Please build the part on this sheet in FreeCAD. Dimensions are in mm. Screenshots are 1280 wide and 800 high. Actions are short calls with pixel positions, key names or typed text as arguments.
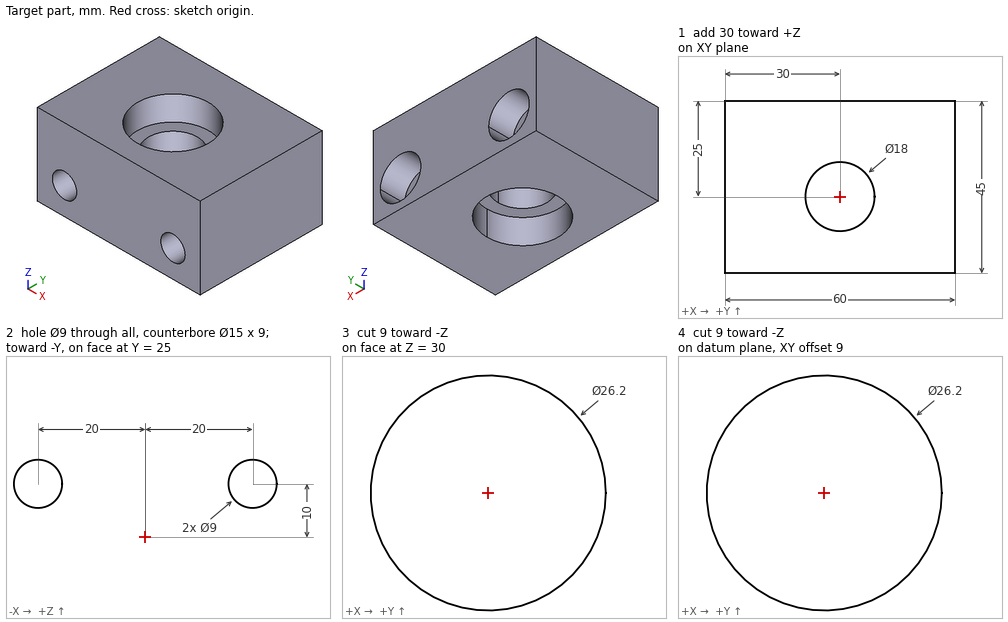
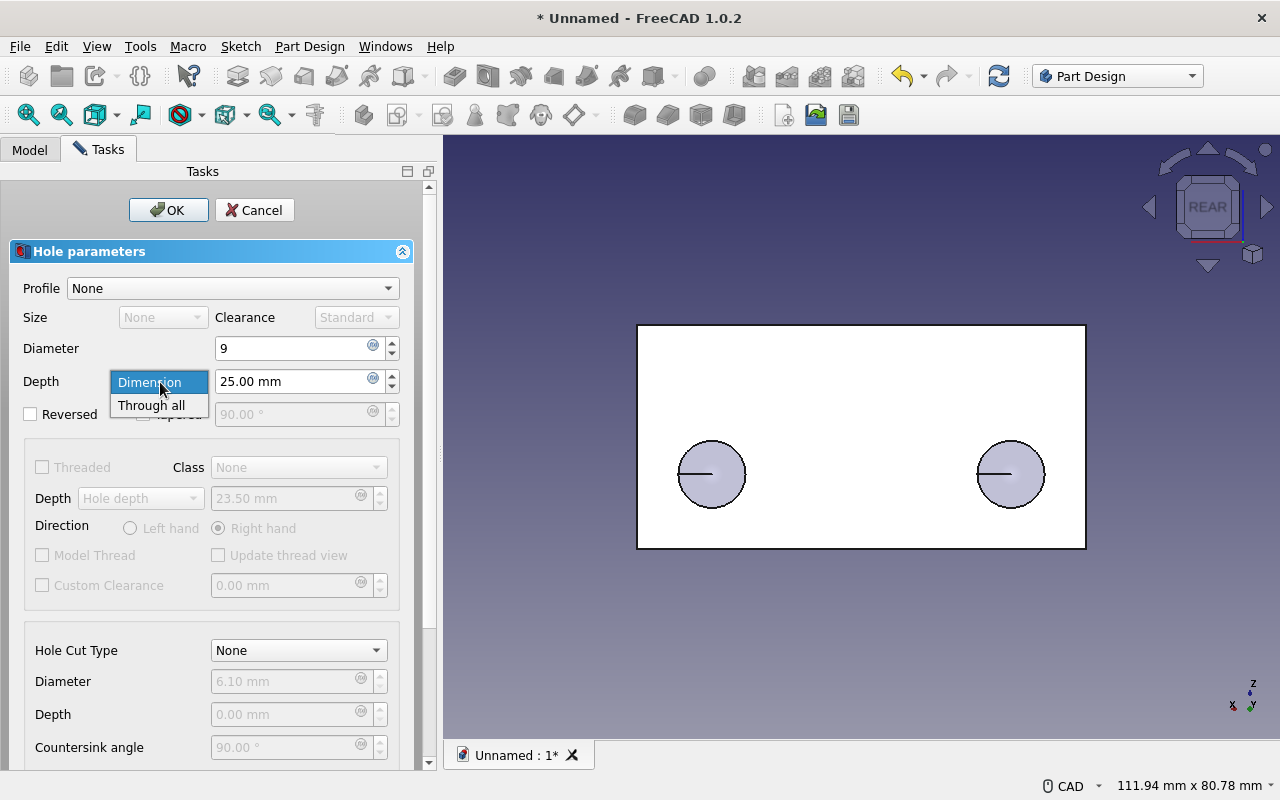
click(158, 406)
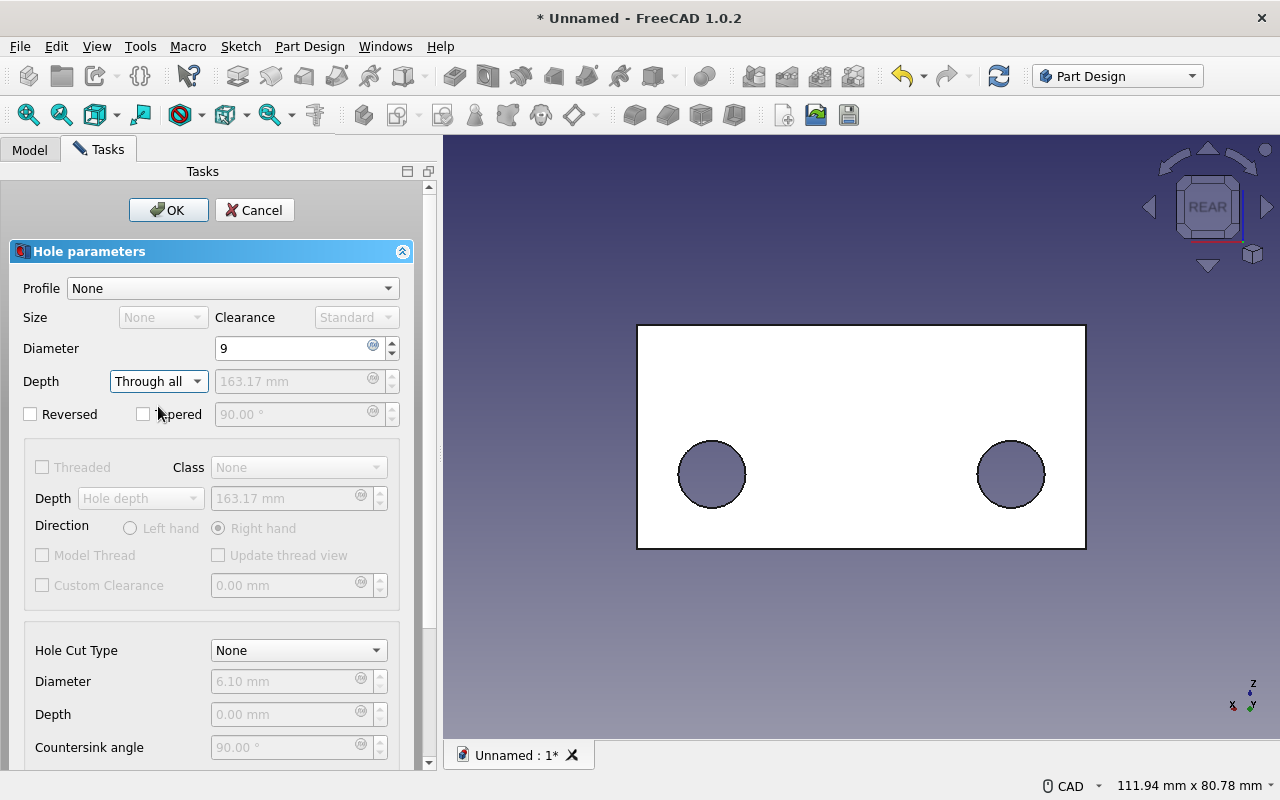
click(300, 650)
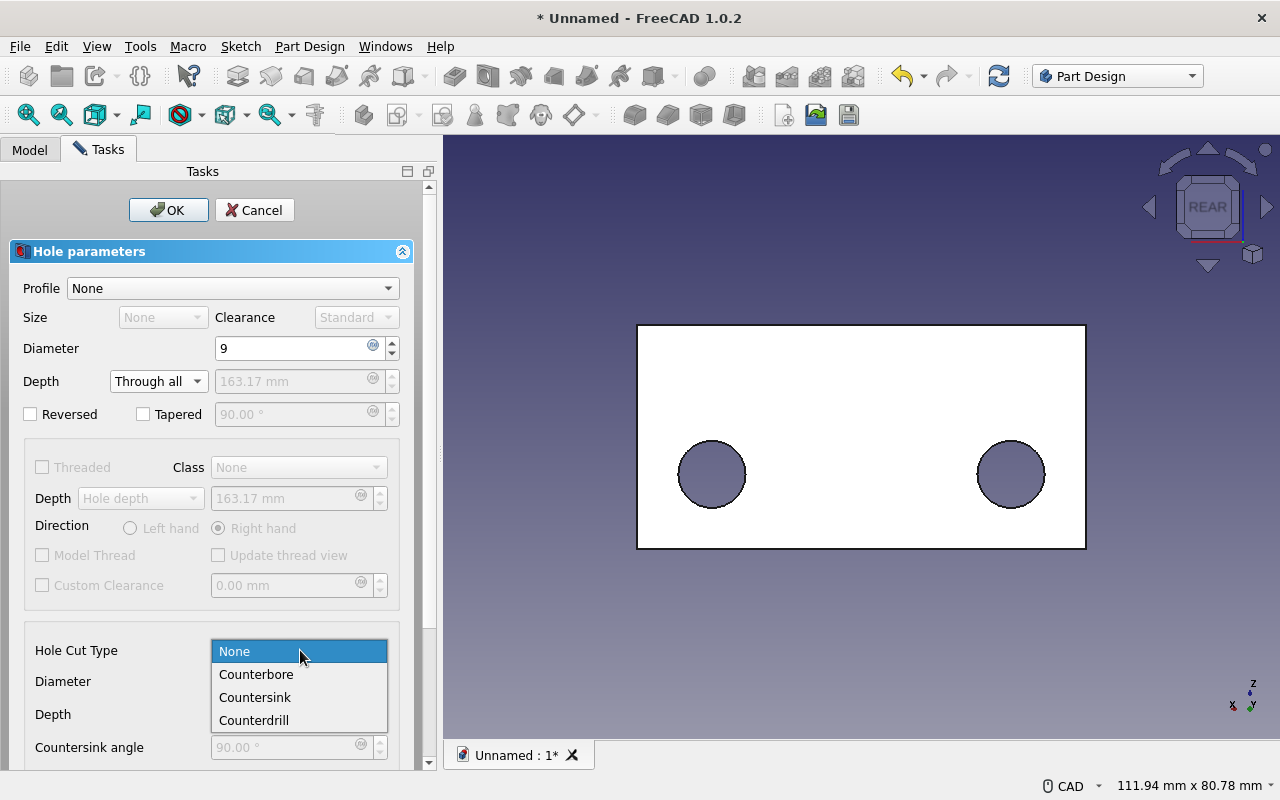
click(298, 674)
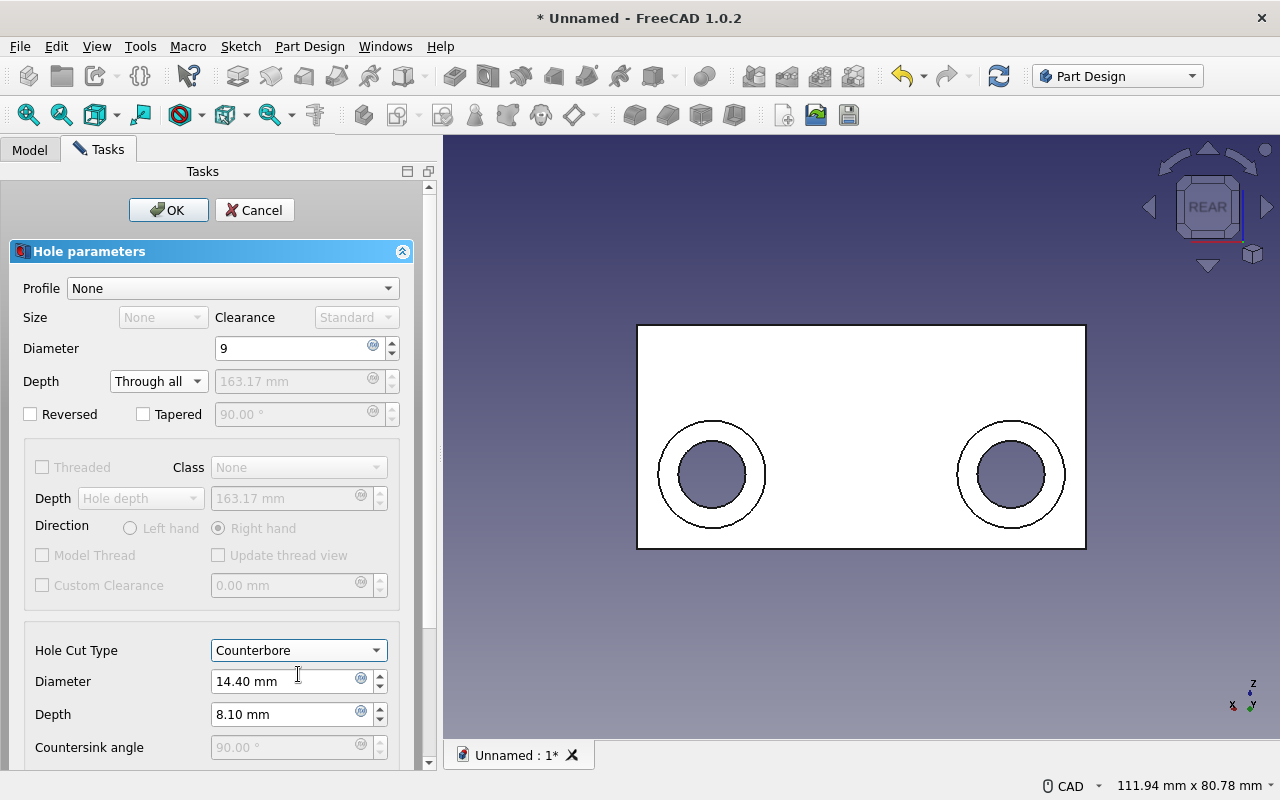
triple_click(292, 682)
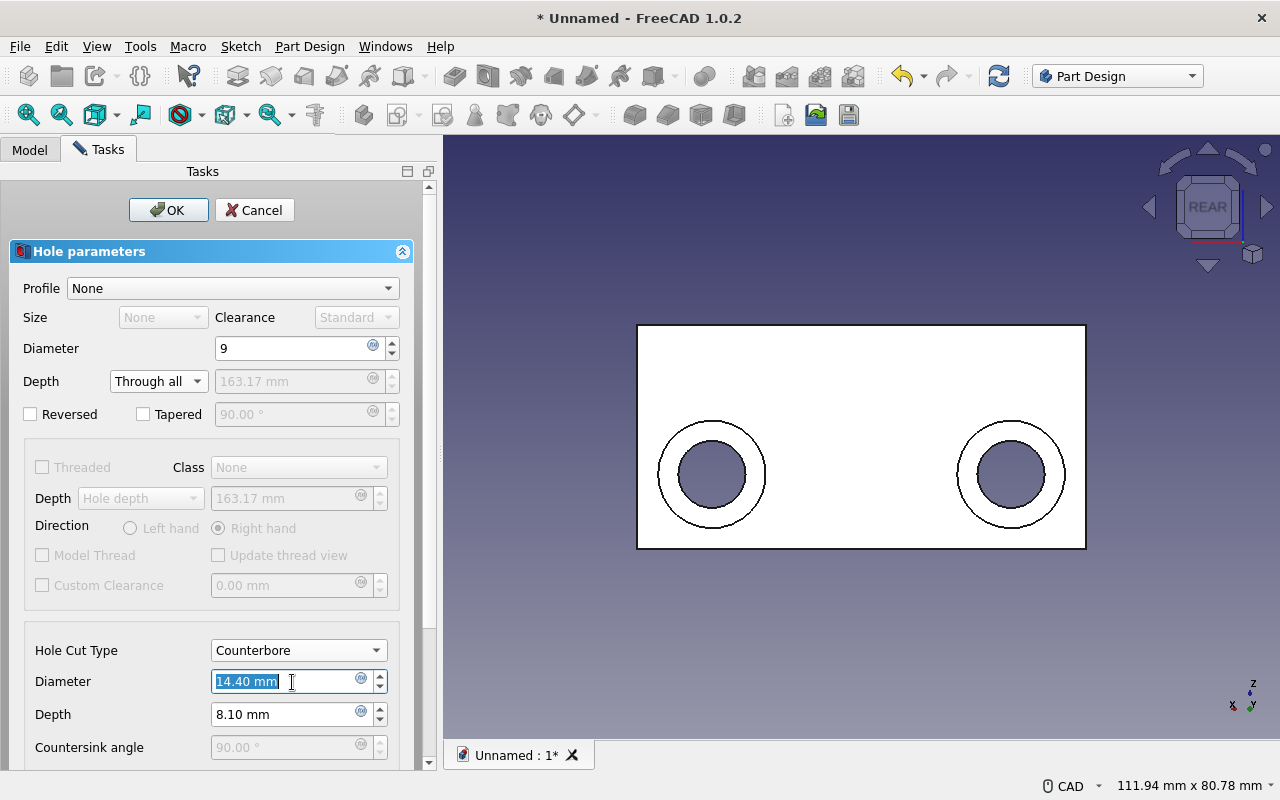
text(15)
key(Tab)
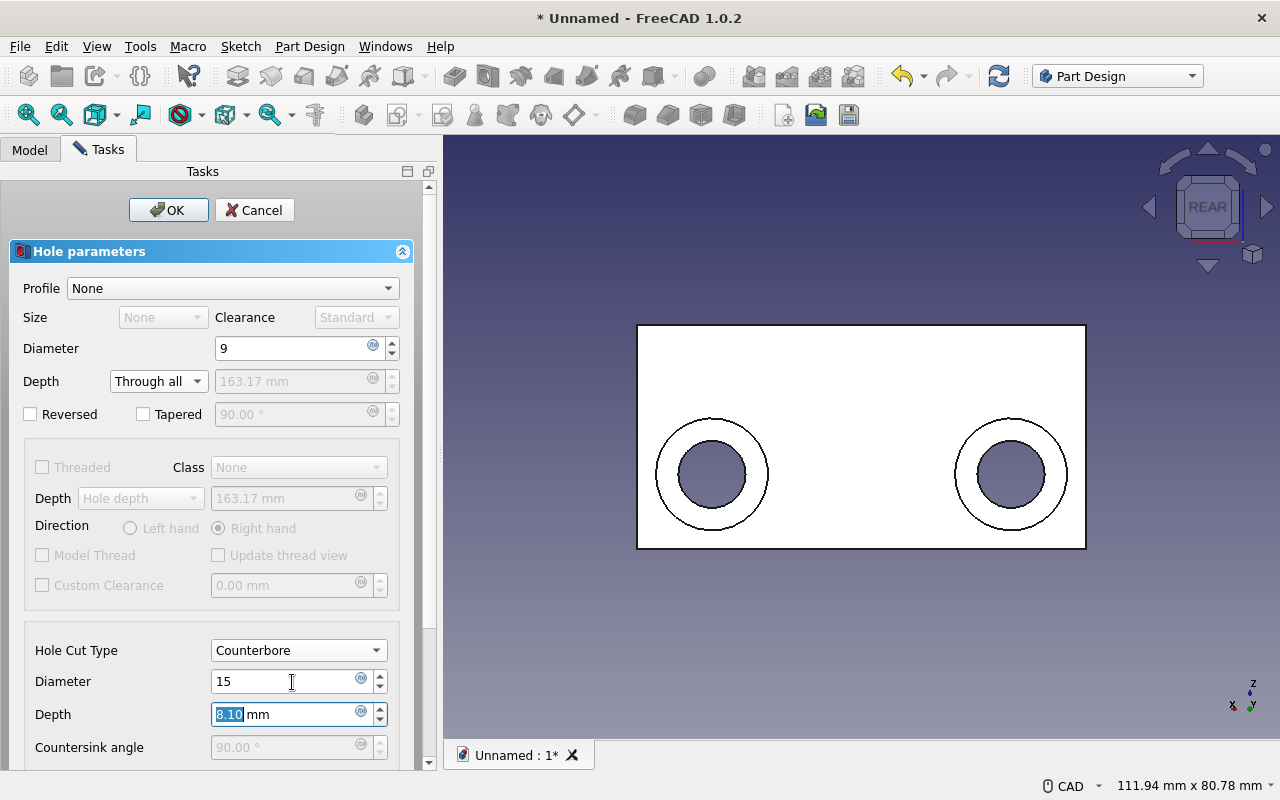
text(9)
key(Tab)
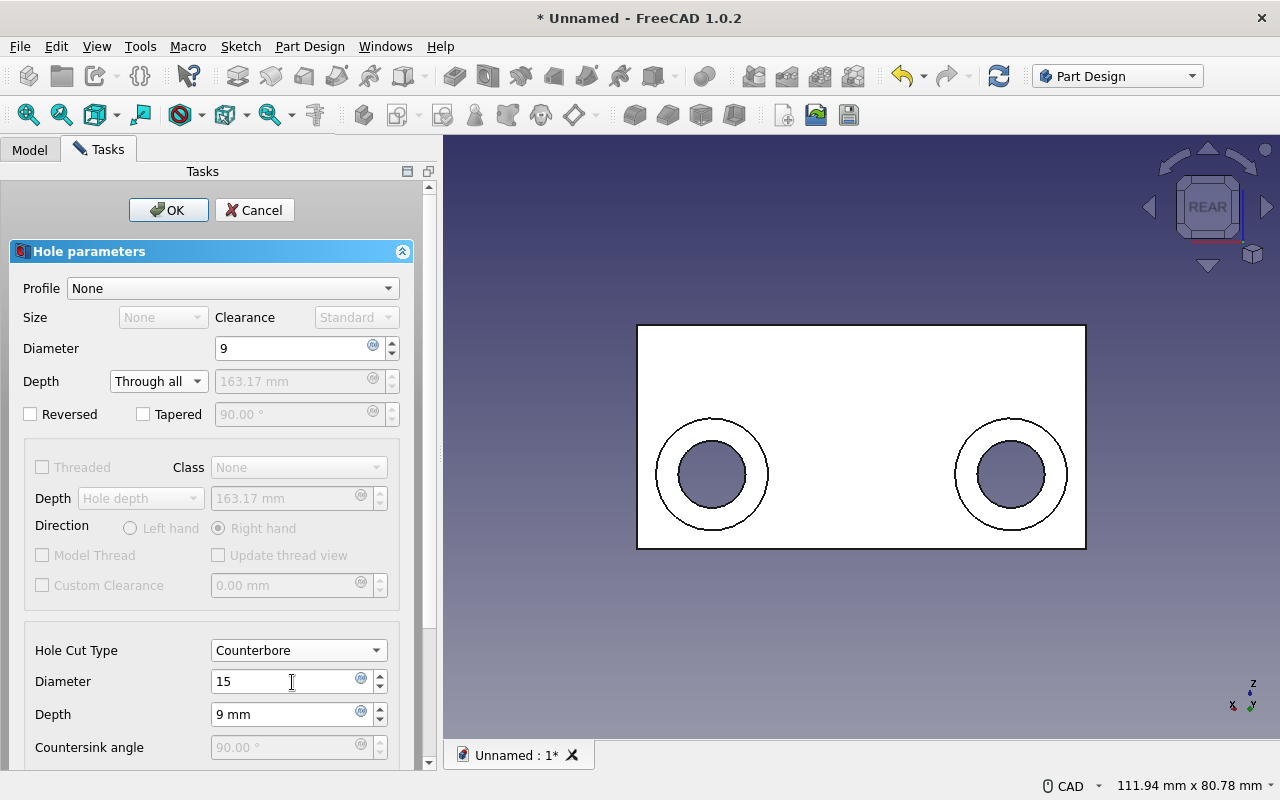
click(169, 210)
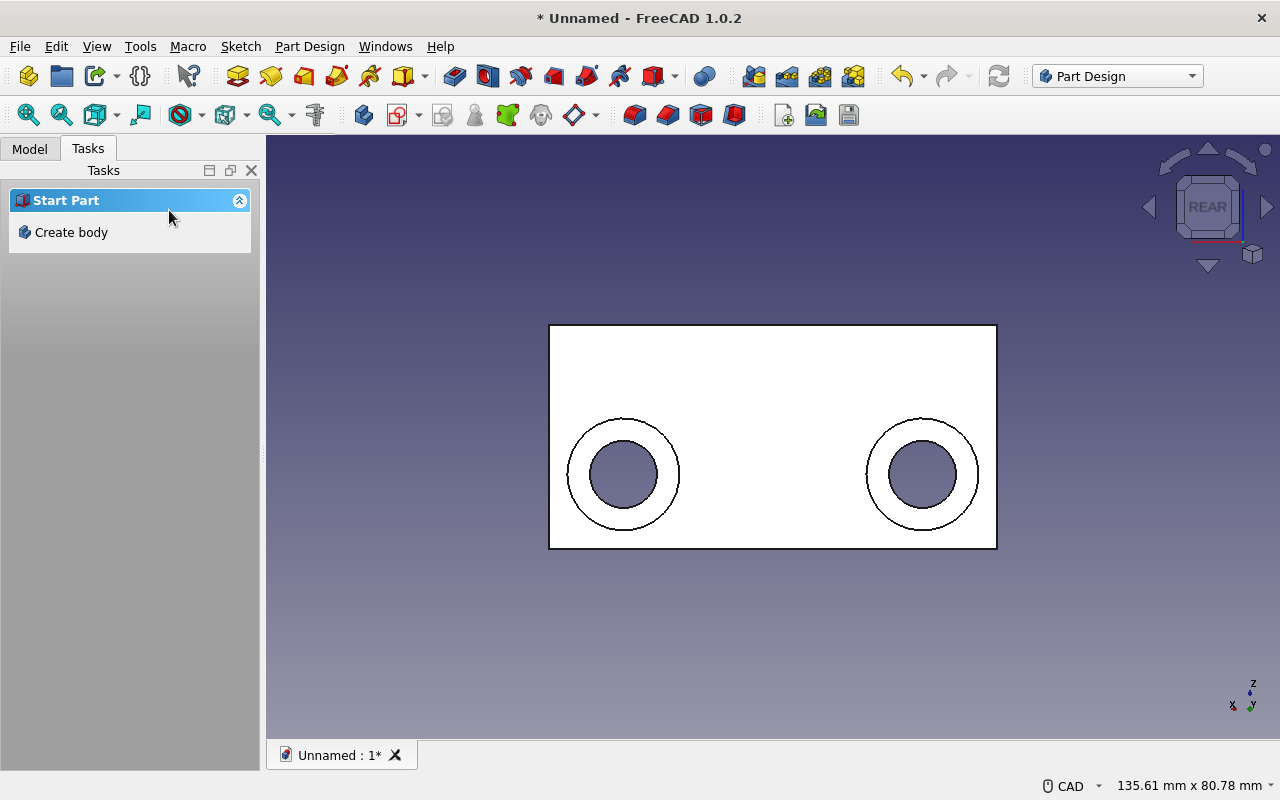
click(29, 116)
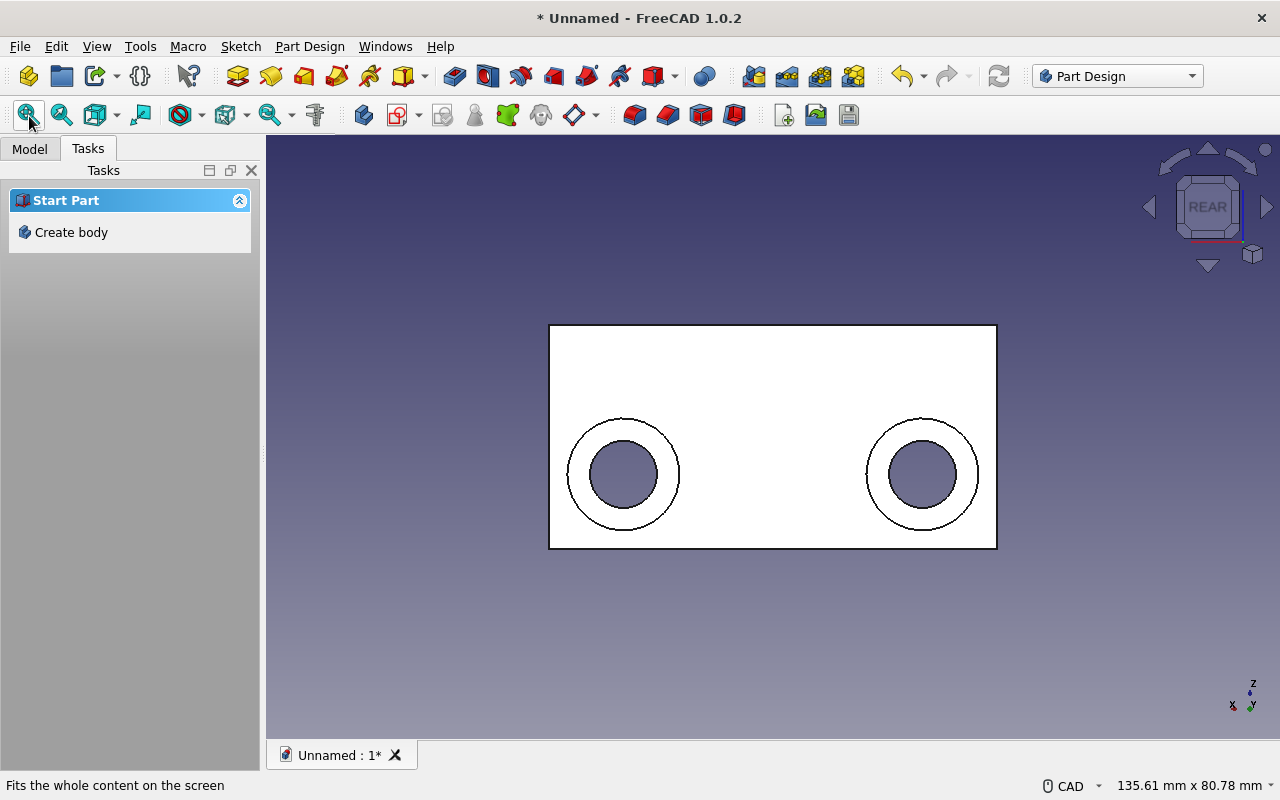
key(0)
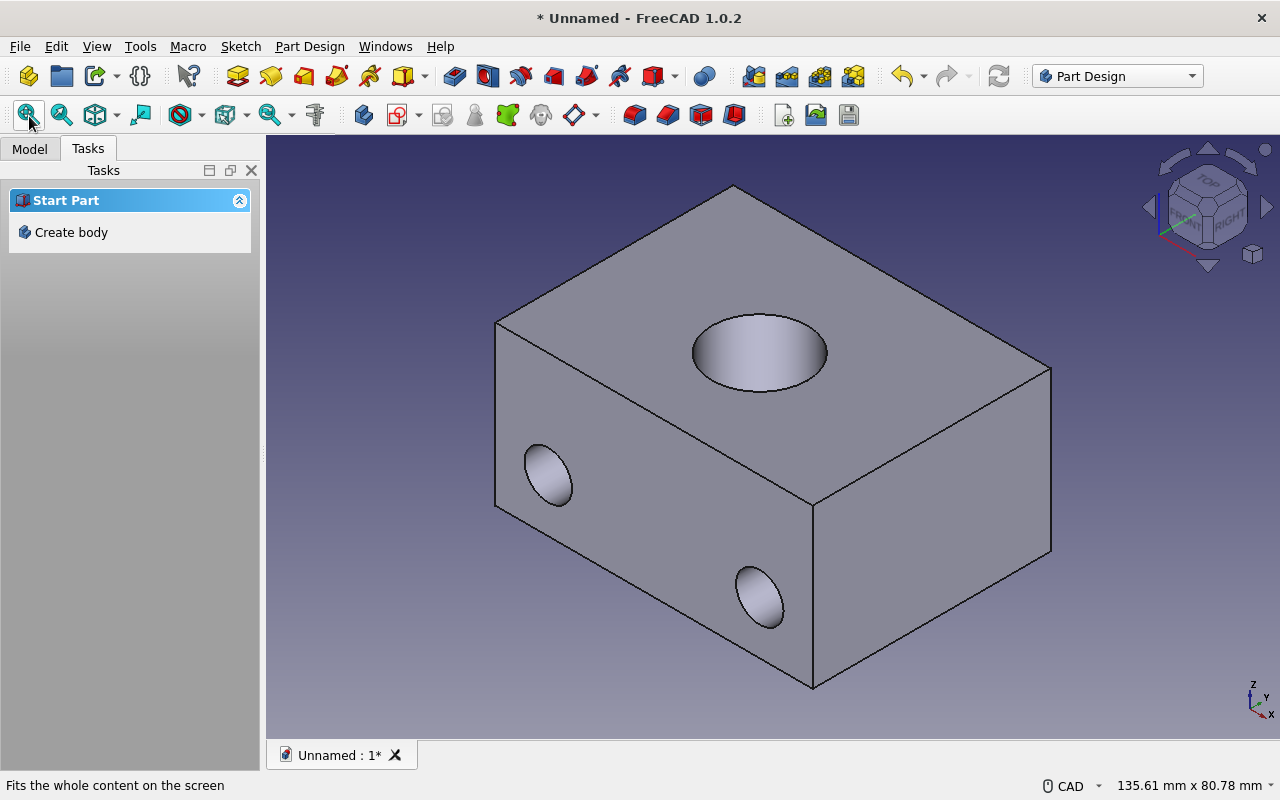
click(898, 377)